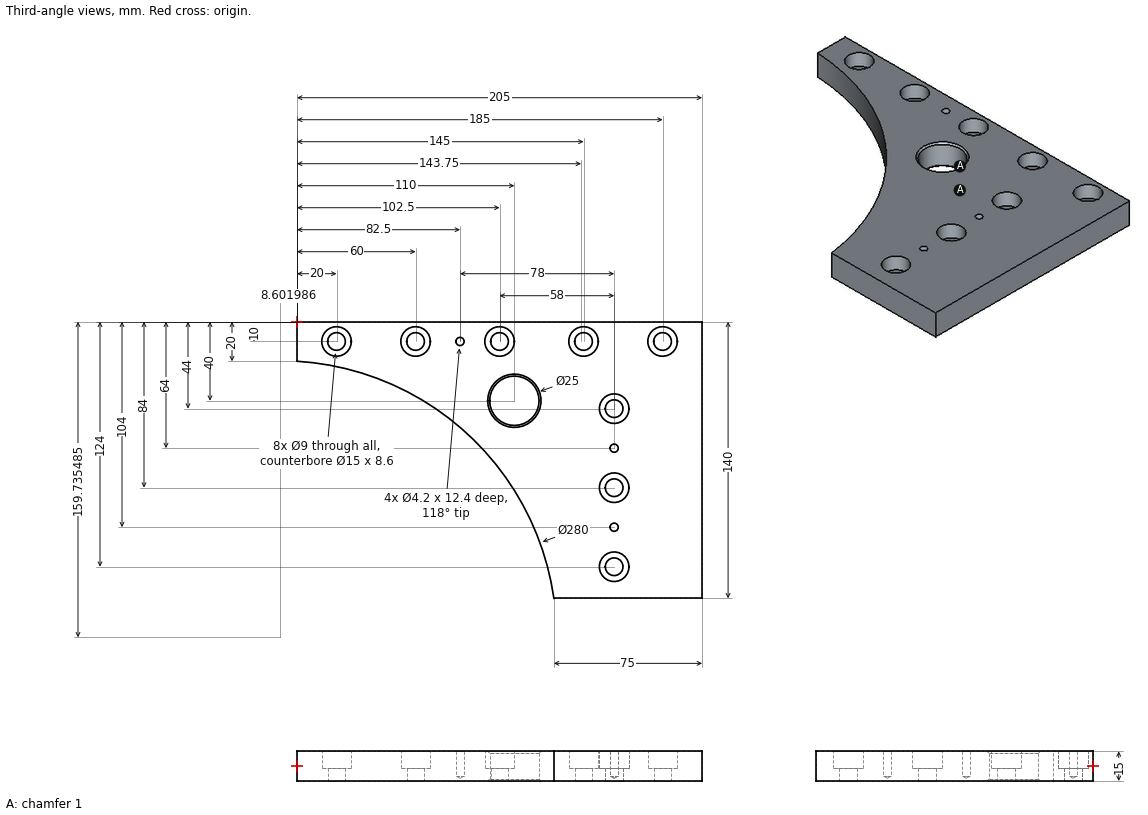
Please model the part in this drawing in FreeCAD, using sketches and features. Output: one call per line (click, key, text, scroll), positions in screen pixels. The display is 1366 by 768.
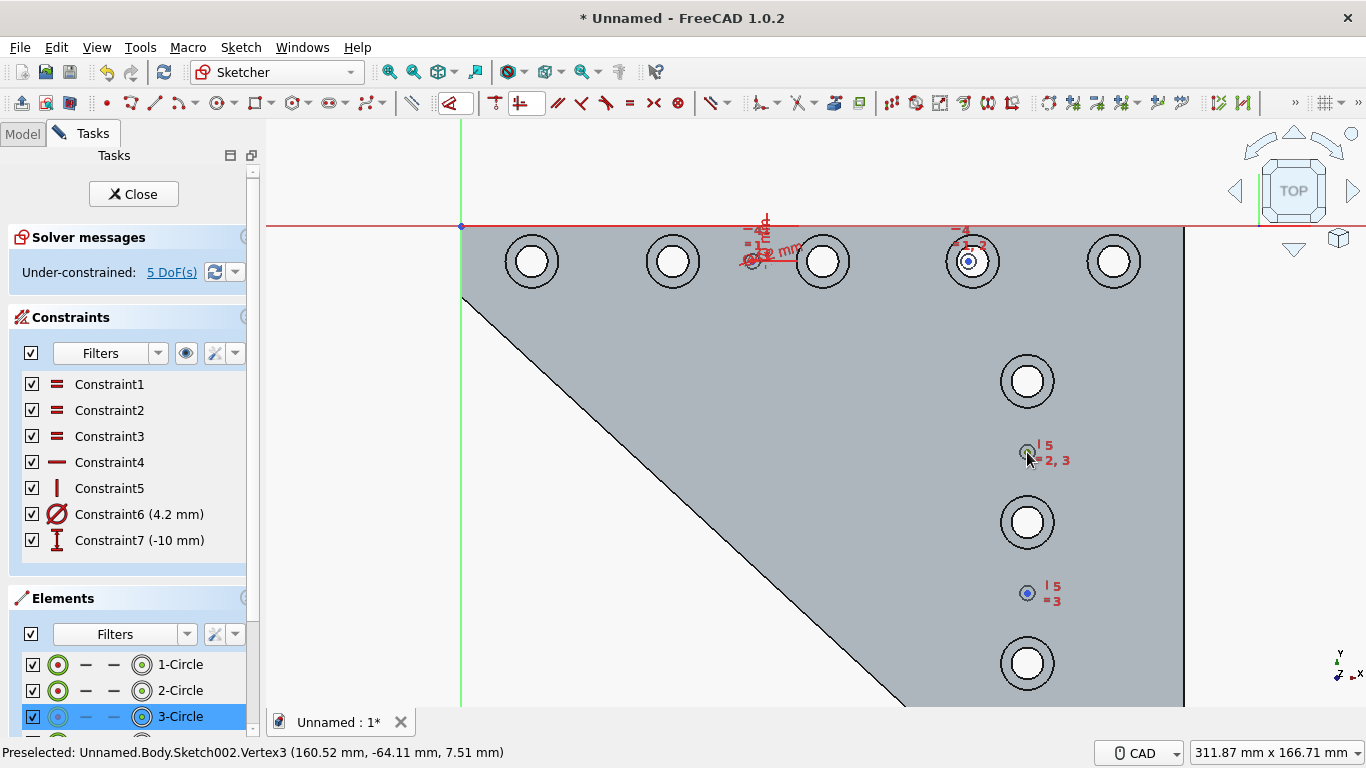
key(i)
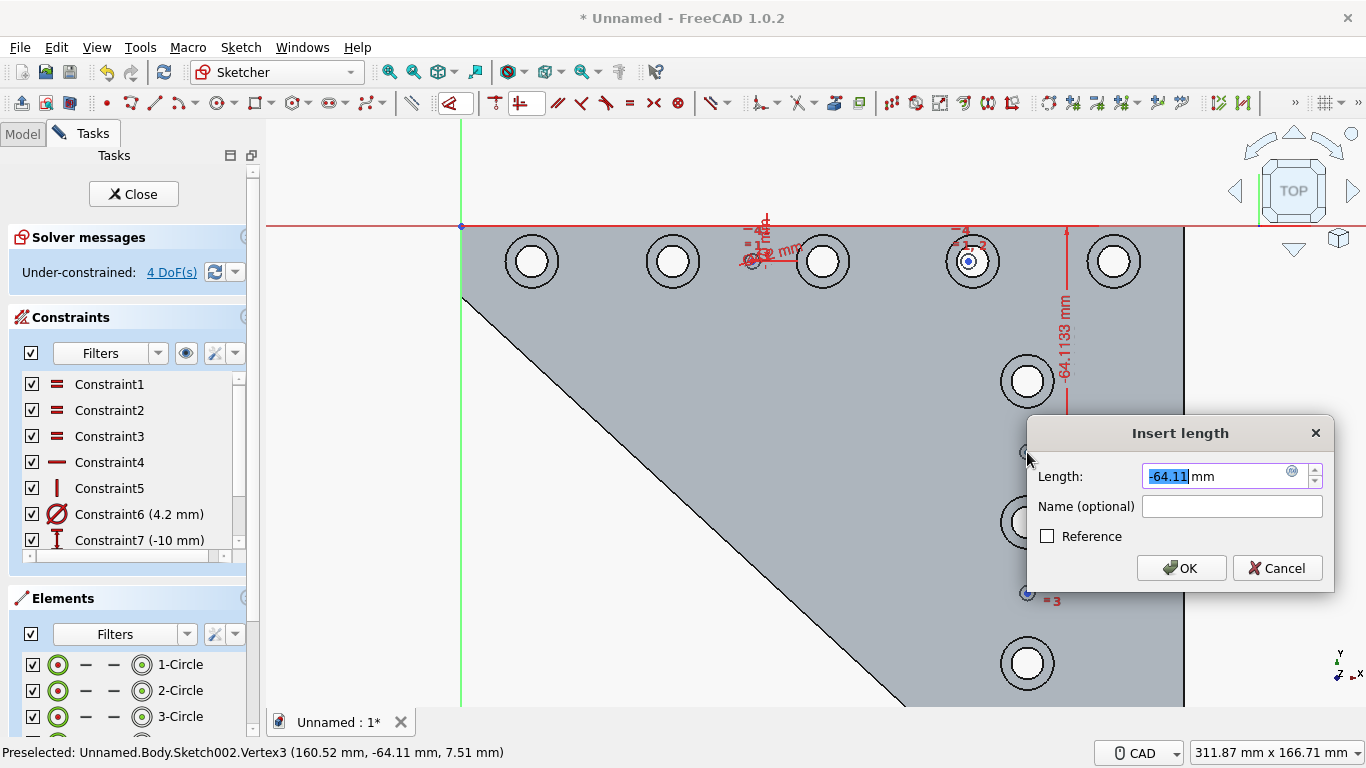
text(-64)
key(Return)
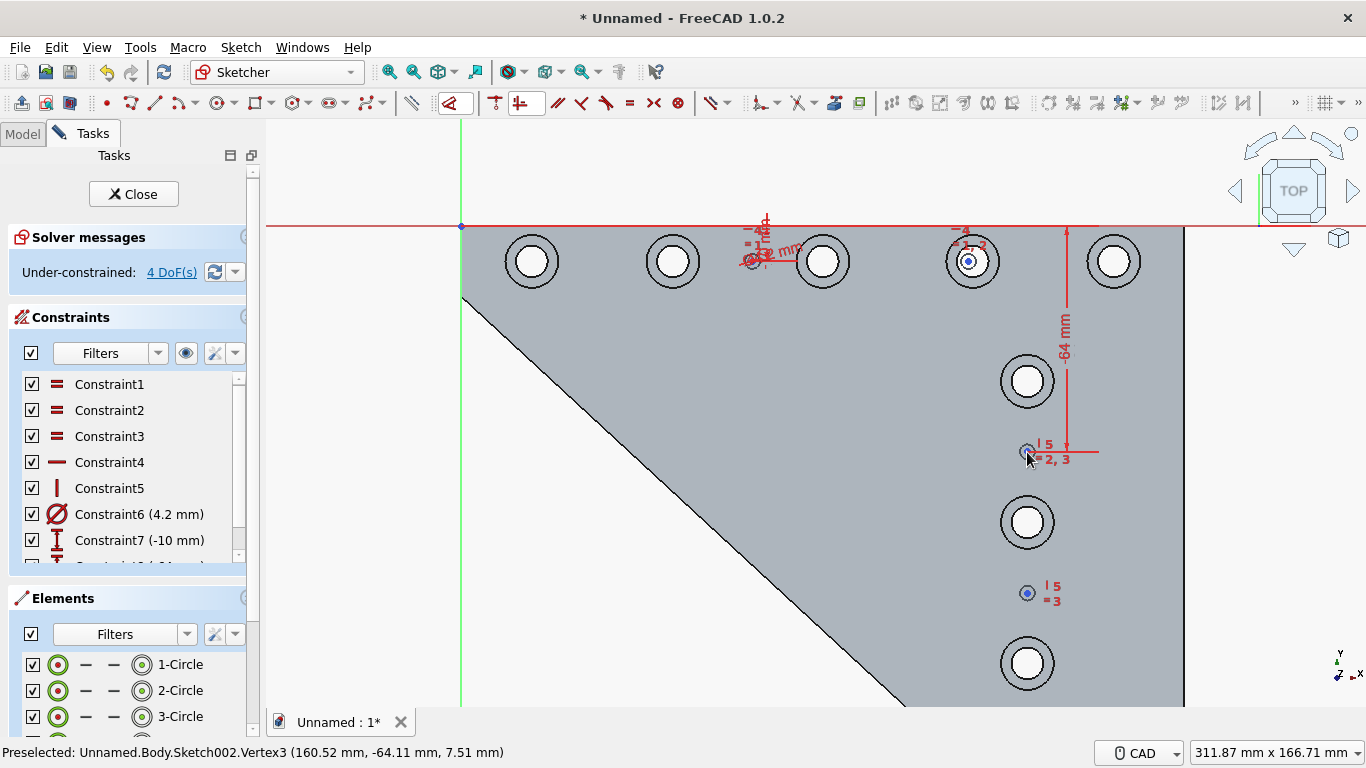
click(1027, 593)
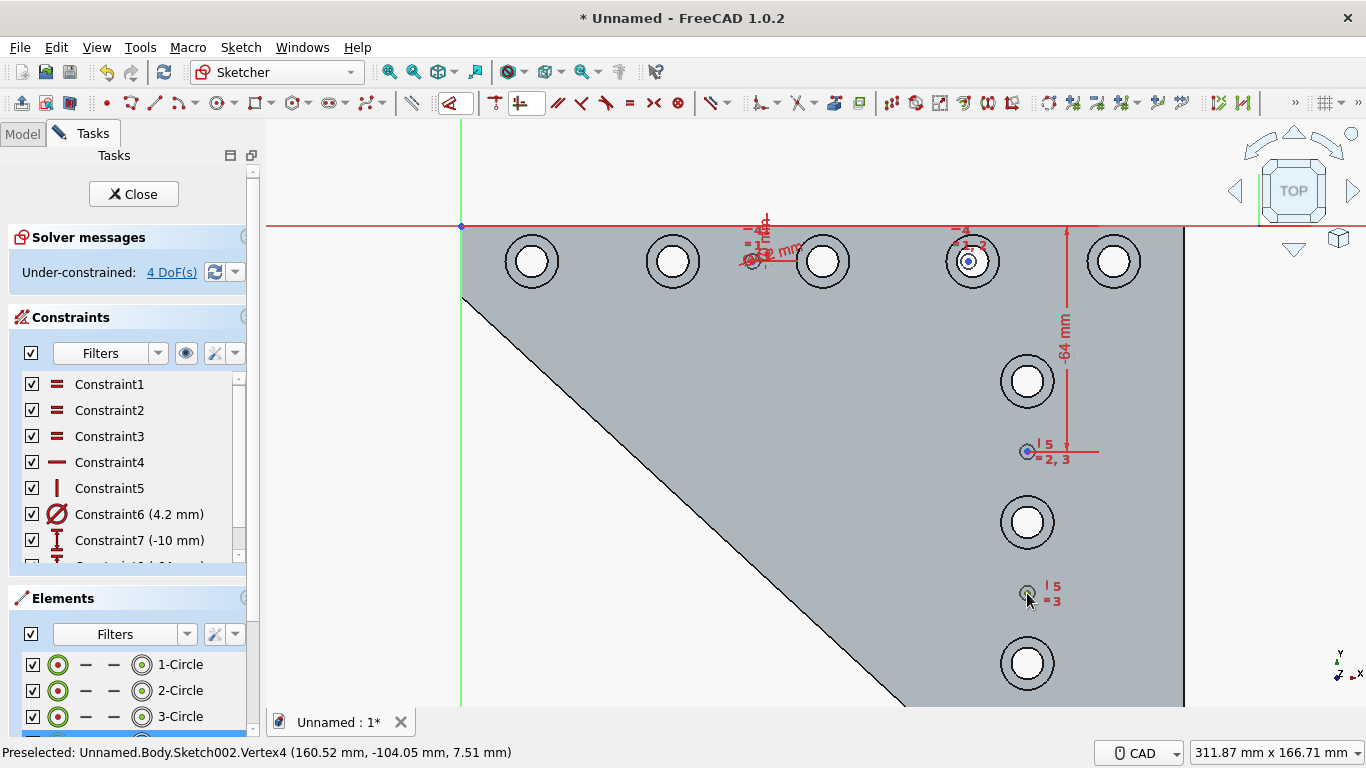
click(468, 104)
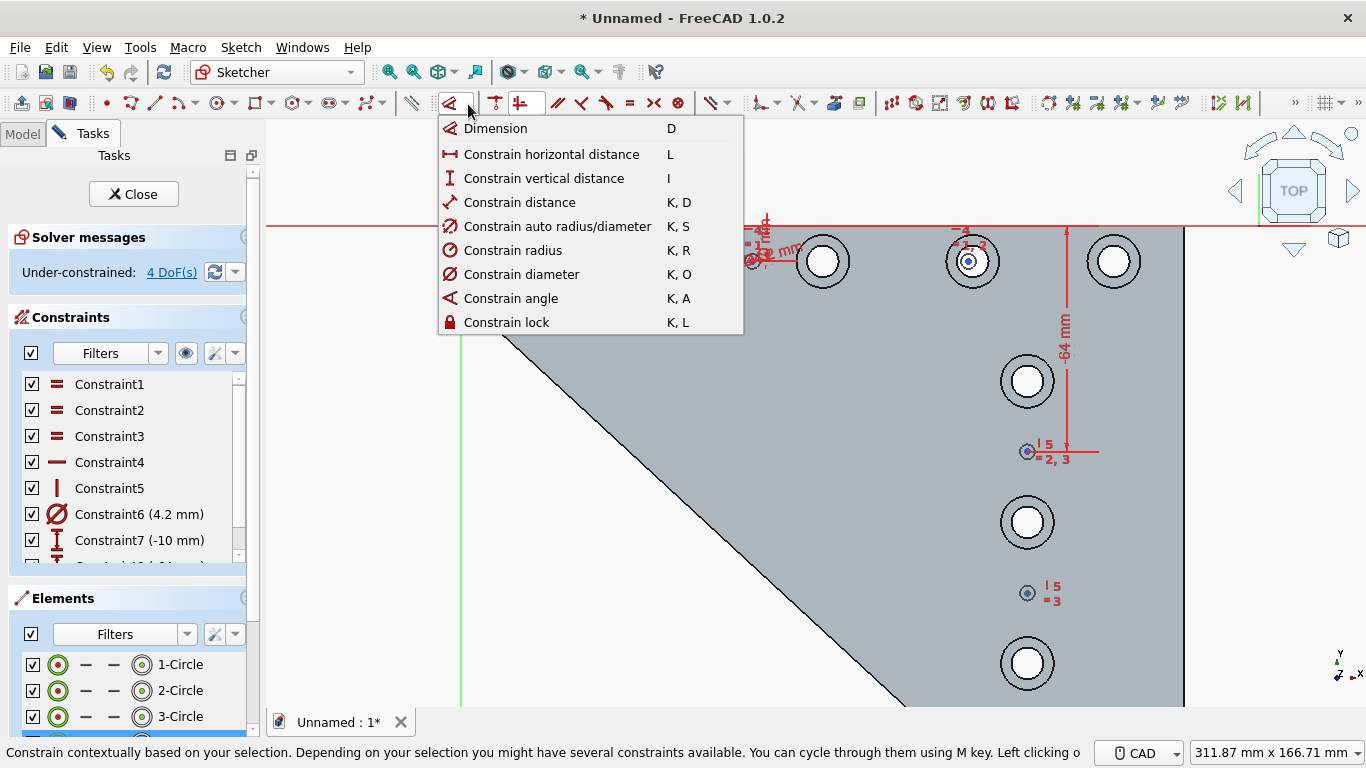
click(591, 178)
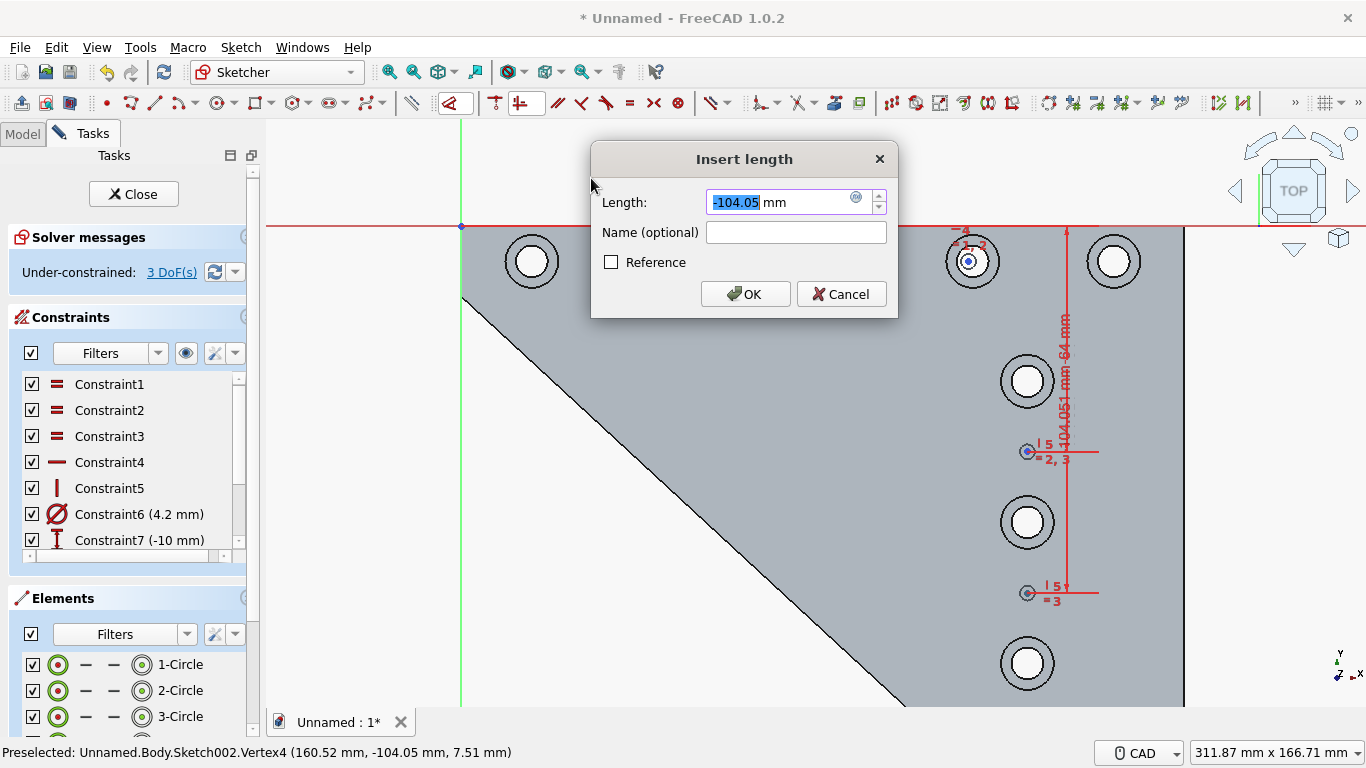
text(-104)
key(Return)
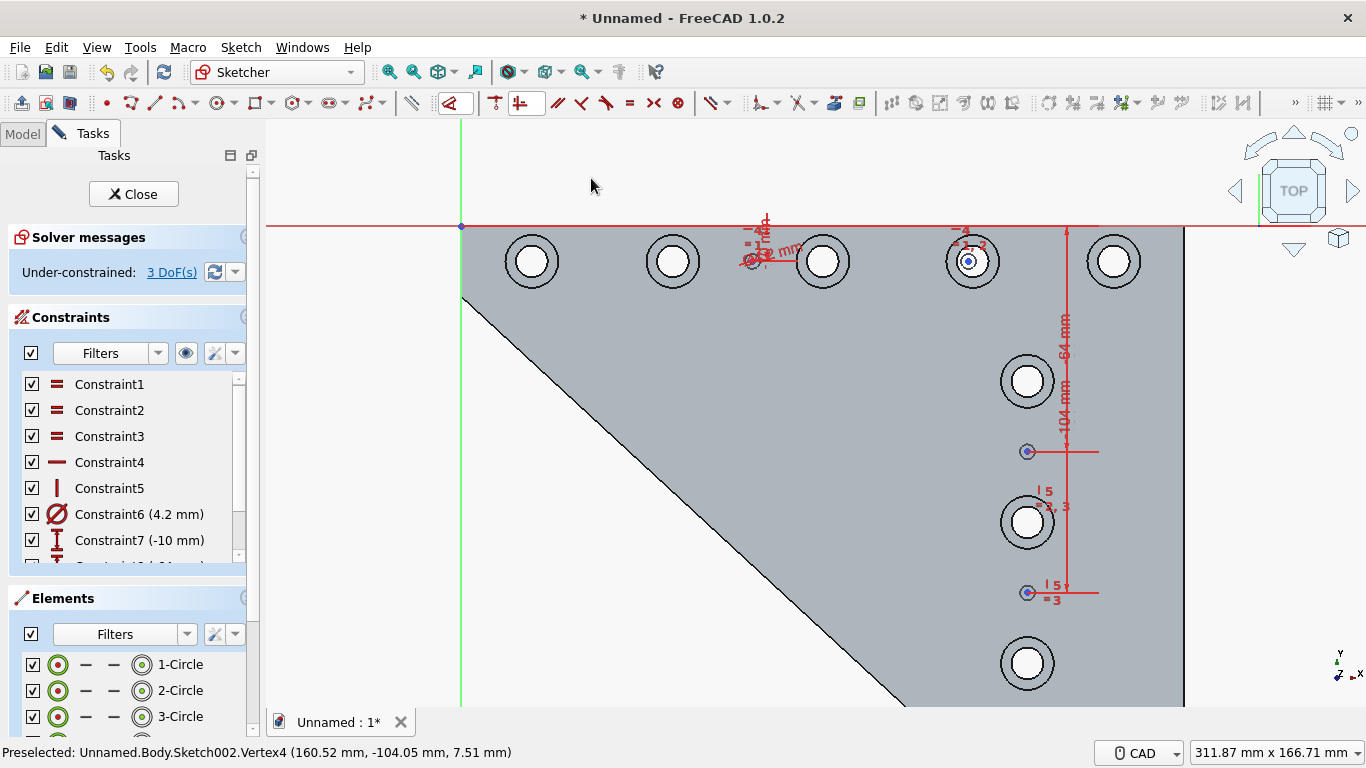
click(752, 261)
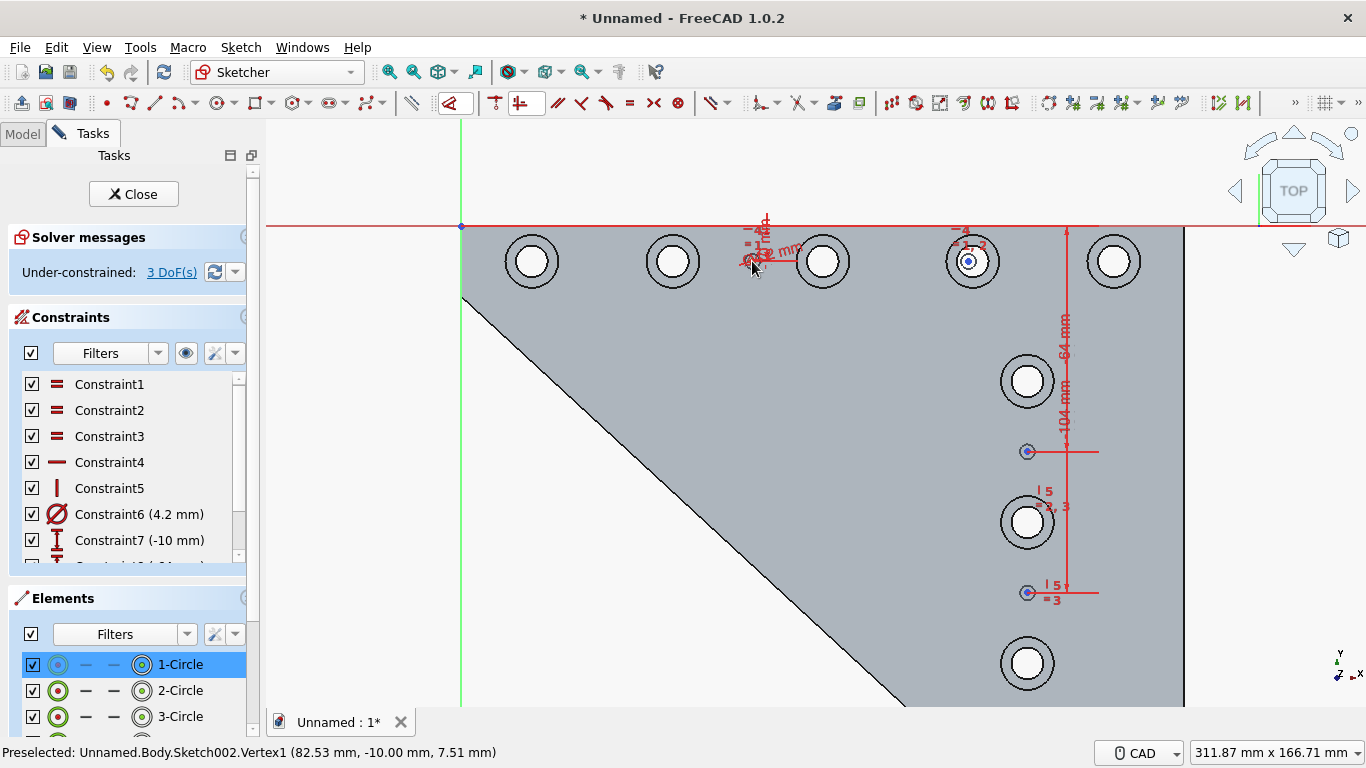
click(1027, 452)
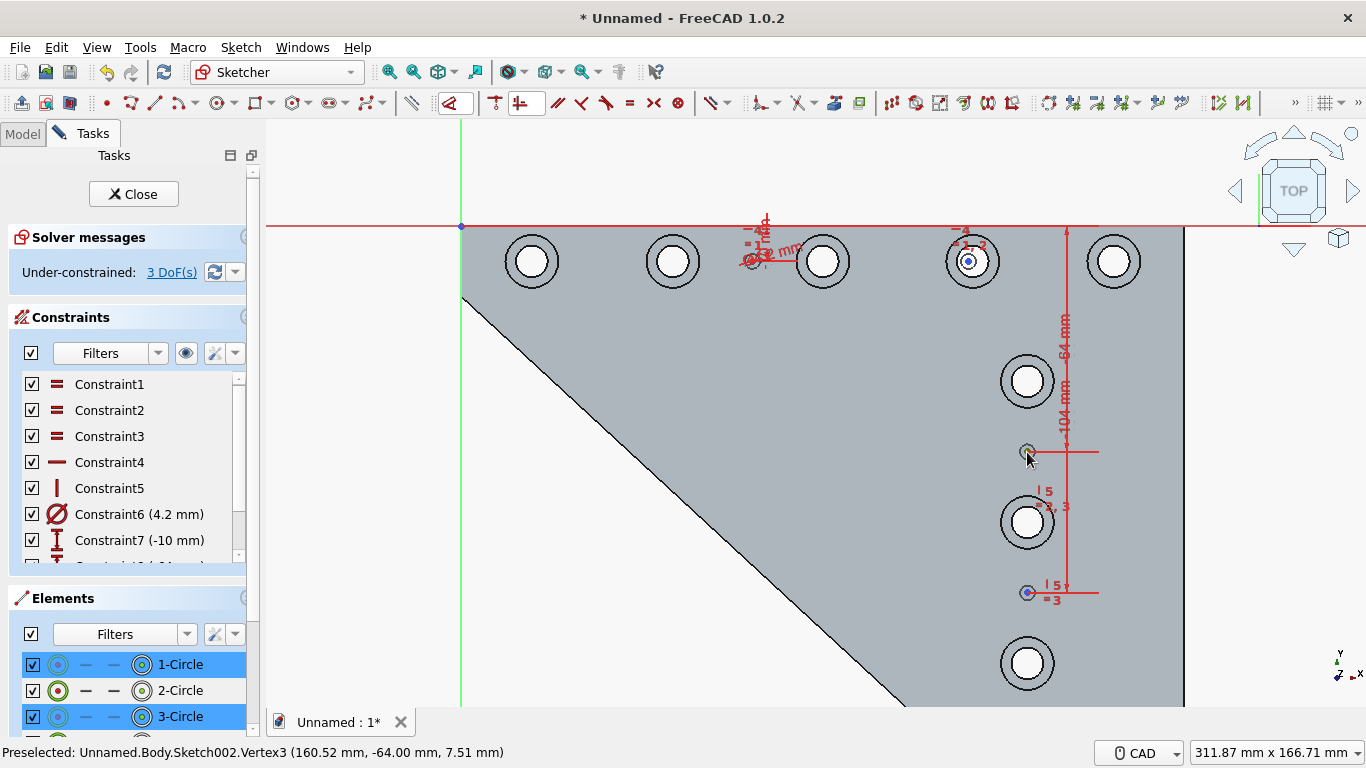
key(l)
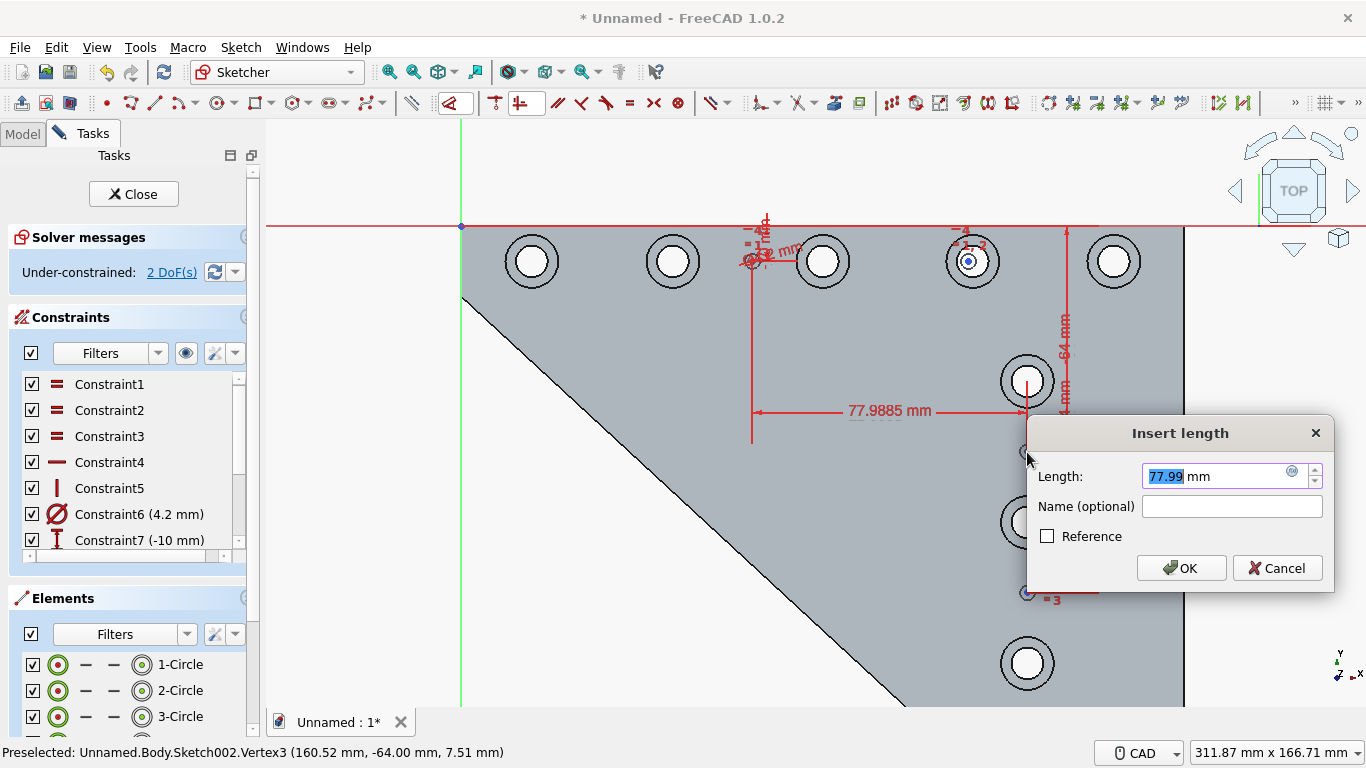
text(78)
key(Return)